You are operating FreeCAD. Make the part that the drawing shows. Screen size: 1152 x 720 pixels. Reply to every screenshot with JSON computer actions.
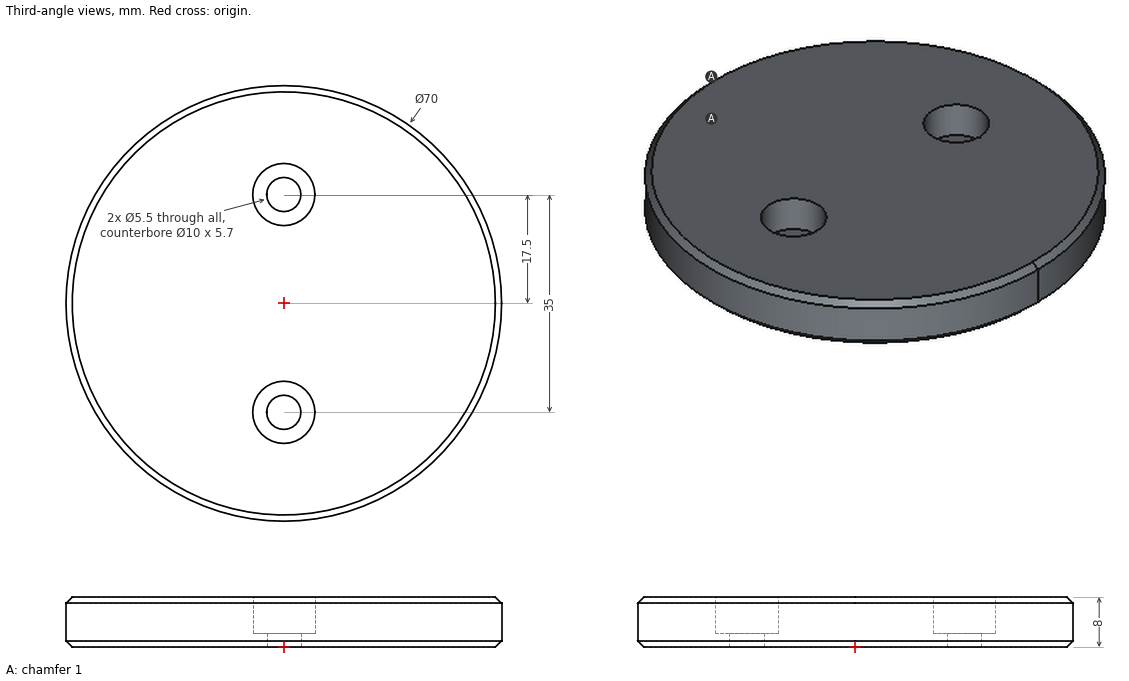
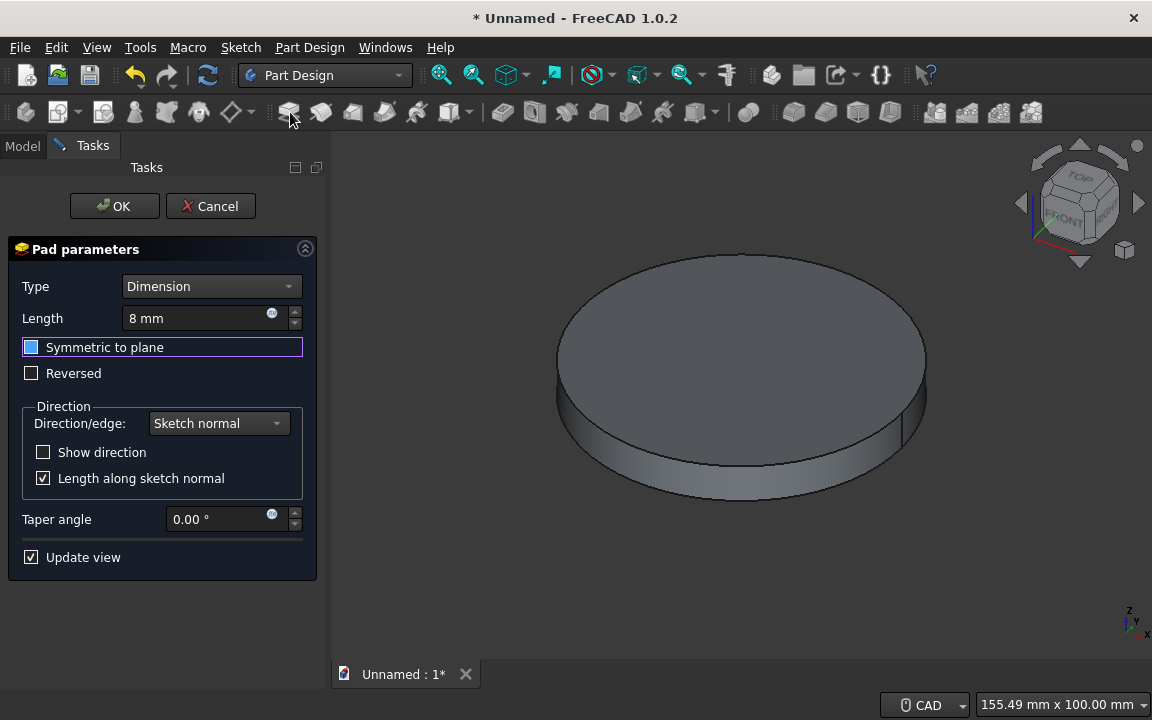
{"action": "left_click", "coordinate": [115, 206]}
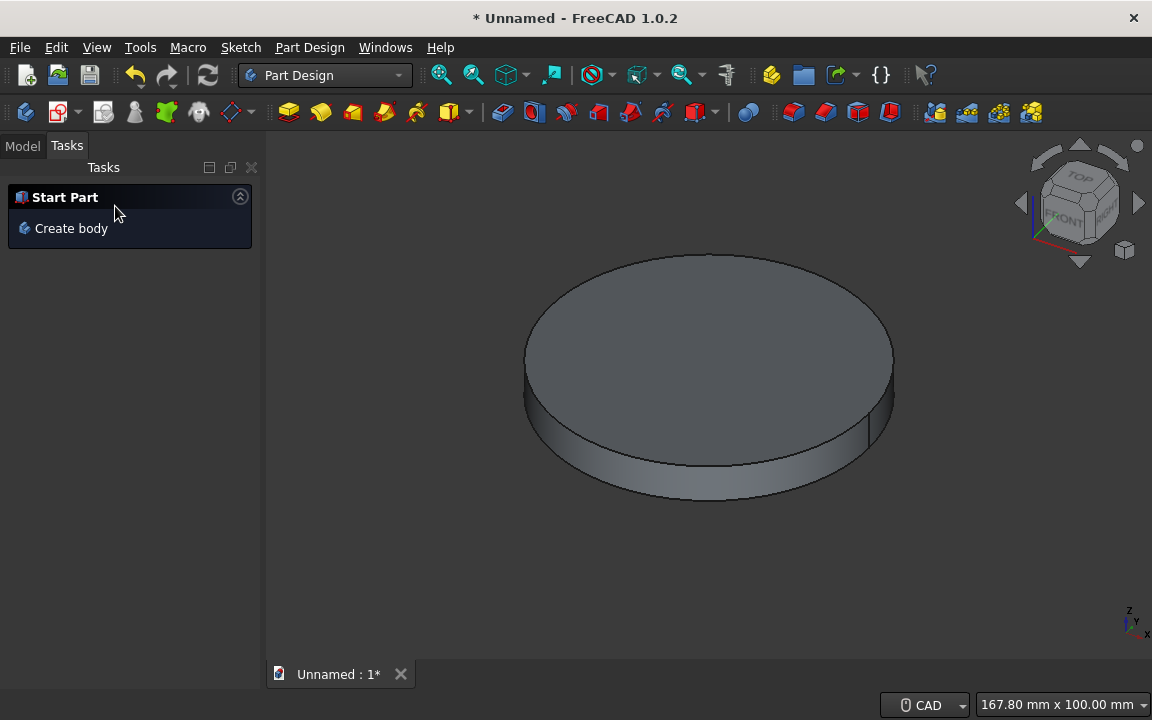
{"action": "left_click", "coordinate": [709, 359]}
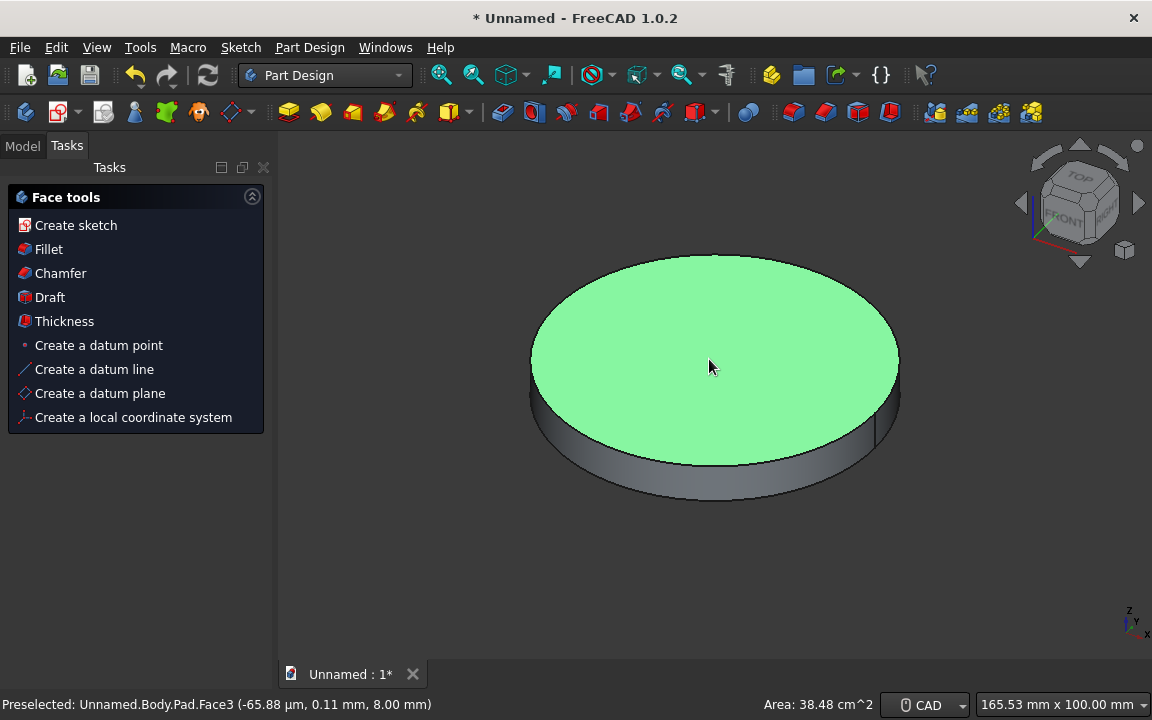
{"action": "left_click", "coordinate": [58, 112]}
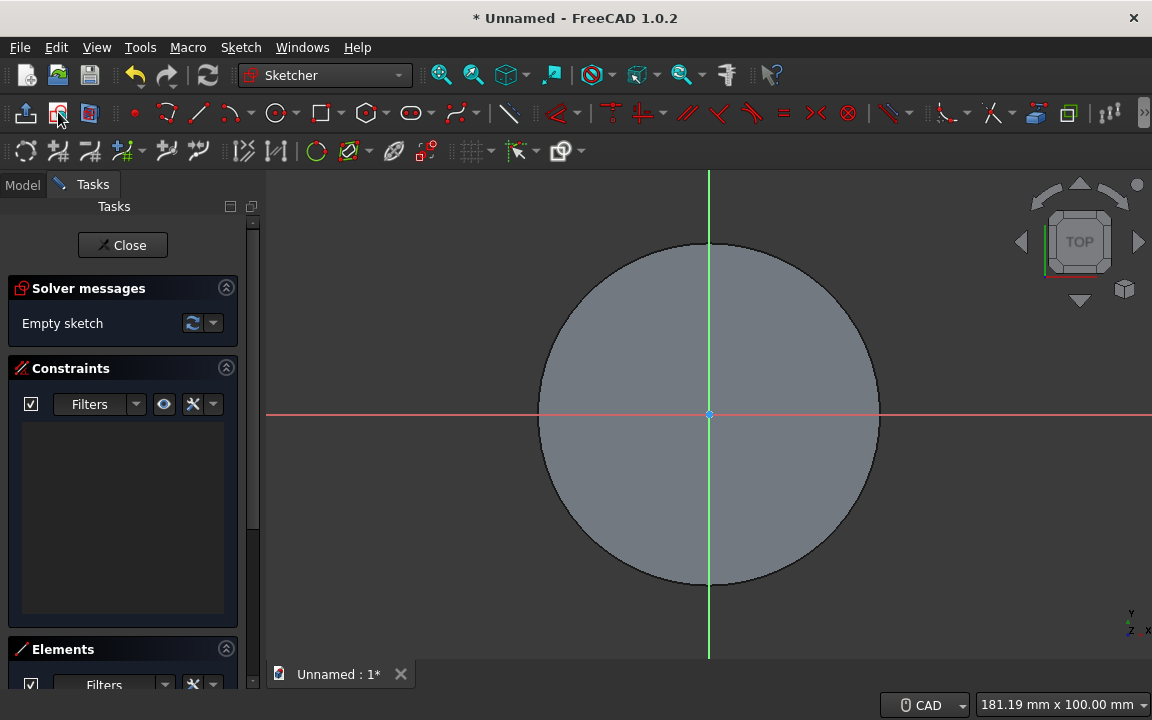
{"action": "scroll", "coordinate": [848, 414], "scroll_direction": "up", "scroll_amount": 2}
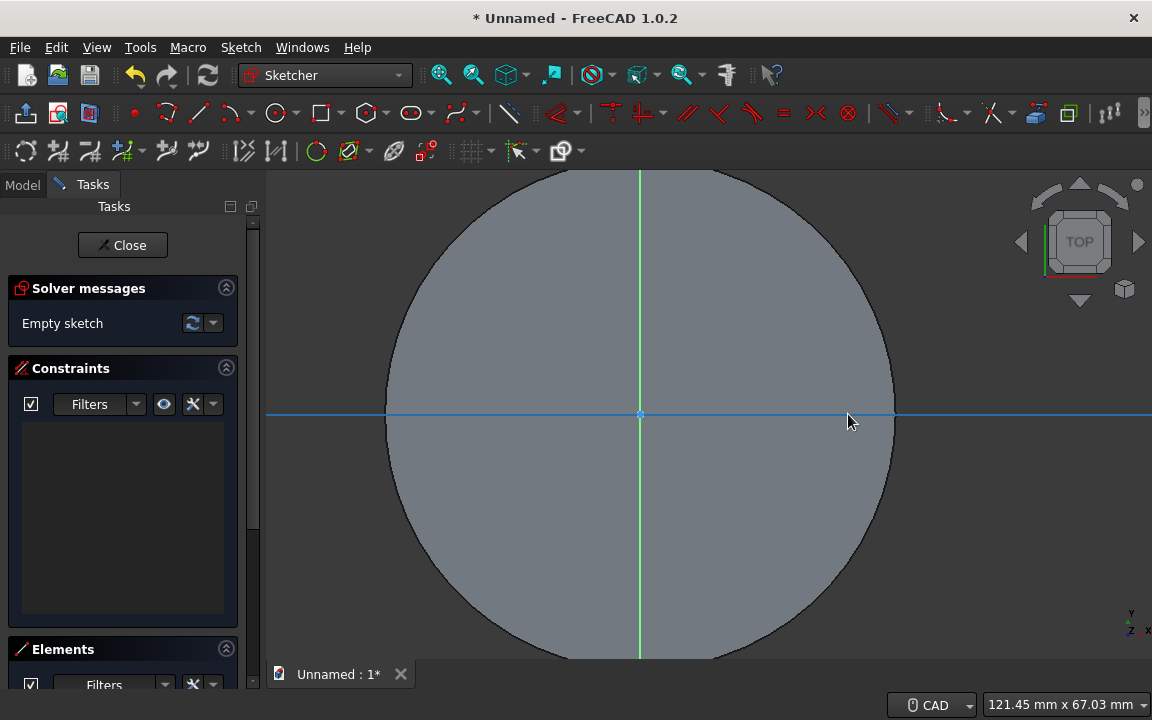
{"action": "left_click", "coordinate": [276, 114]}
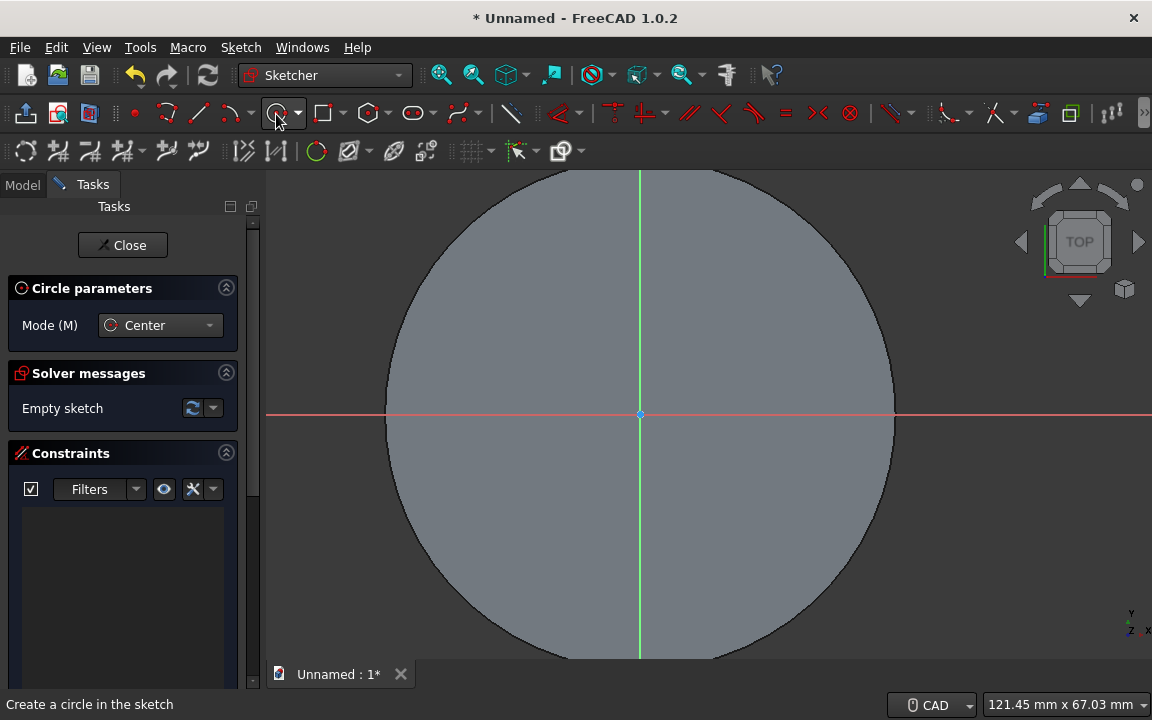
{"action": "left_click", "coordinate": [640, 287]}
{"action": "left_click", "coordinate": [654, 273]}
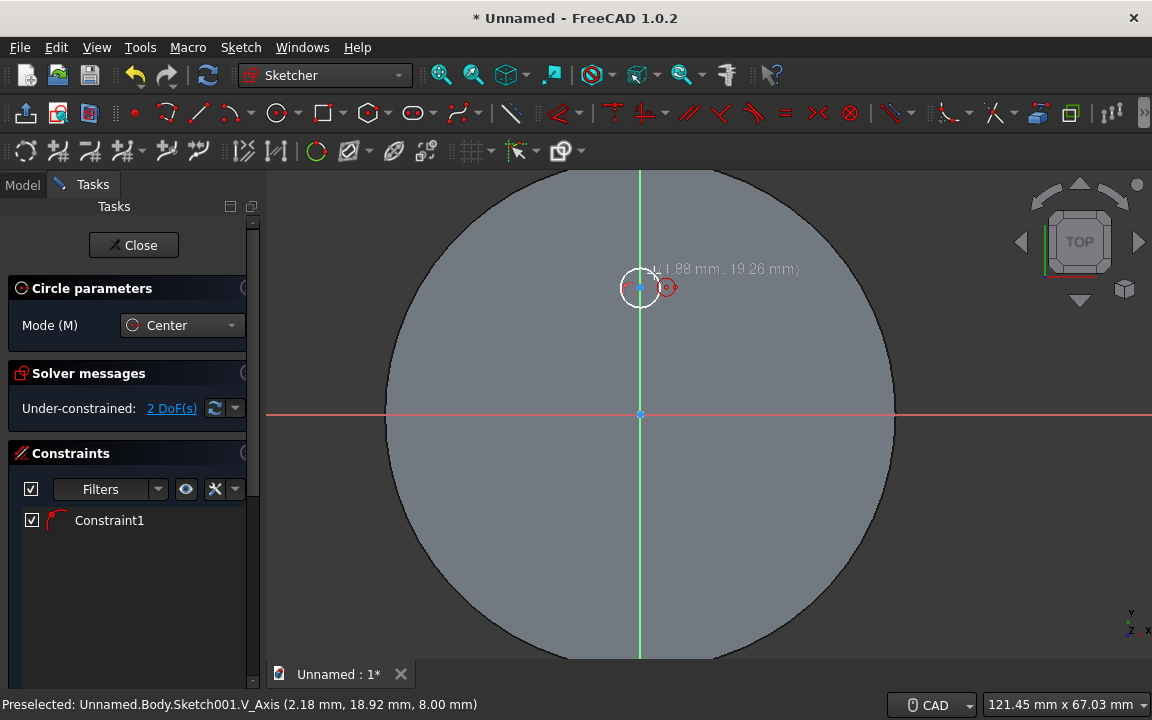
{"action": "left_click", "coordinate": [640, 542]}
{"action": "left_click", "coordinate": [654, 528]}
{"action": "key", "text": "Escape"}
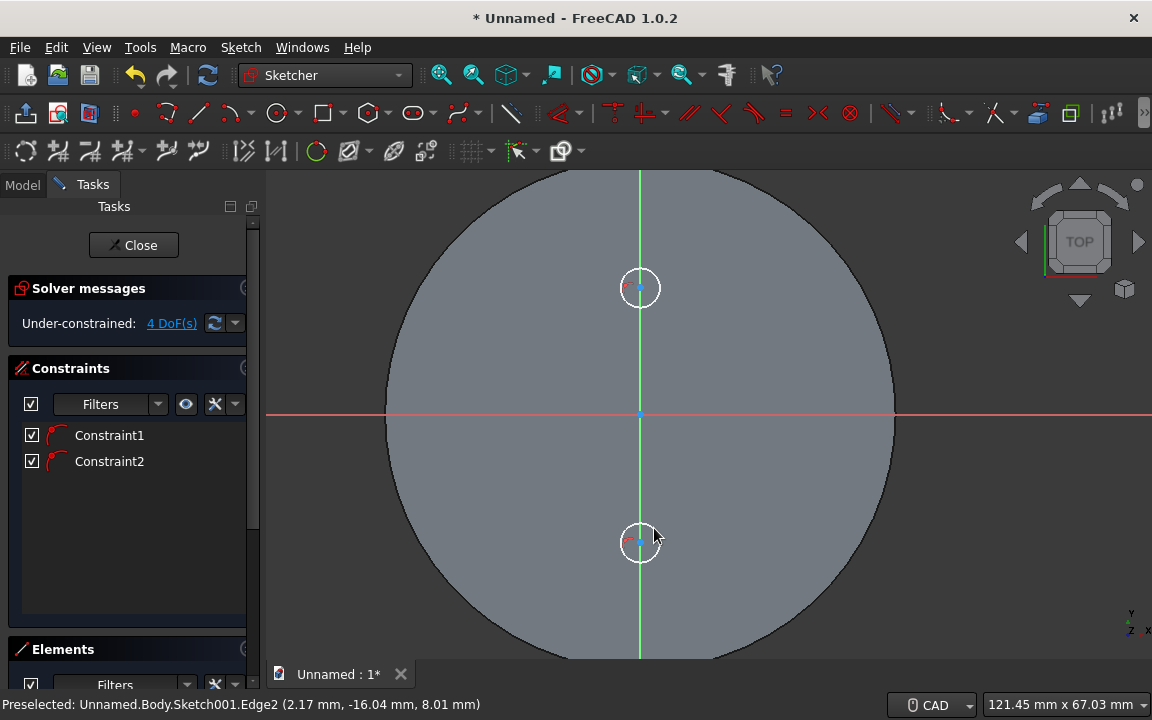
{"action": "left_click", "coordinate": [654, 274]}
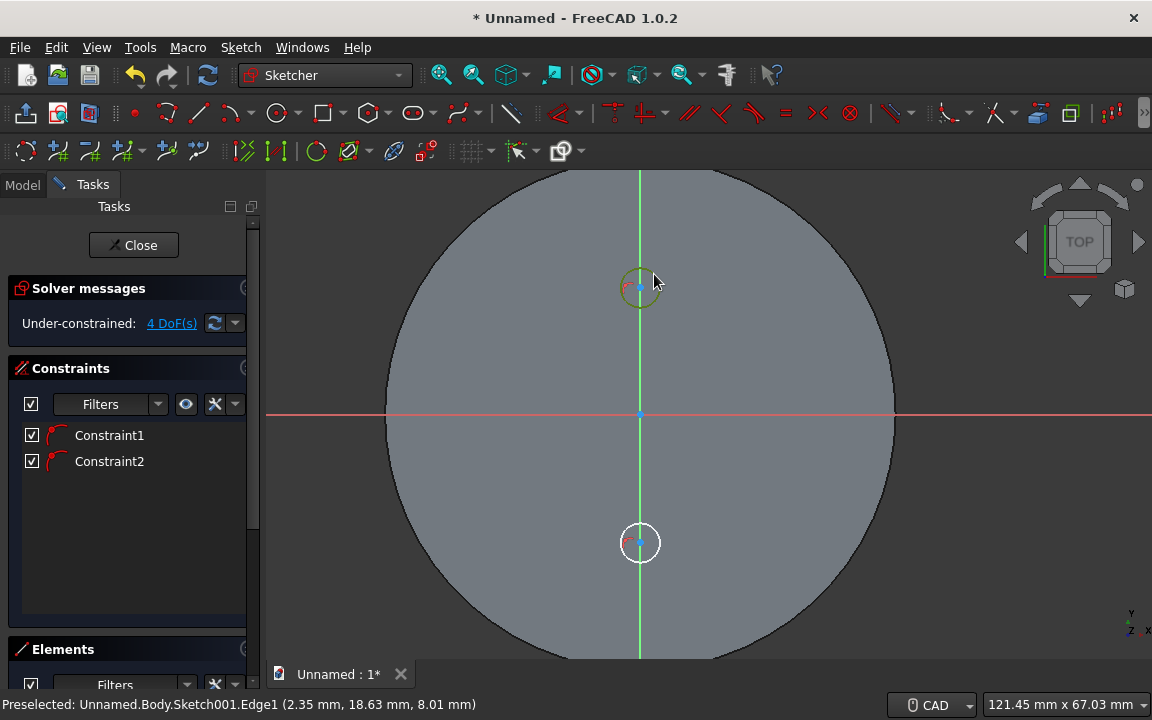
{"action": "left_click", "coordinate": [654, 529]}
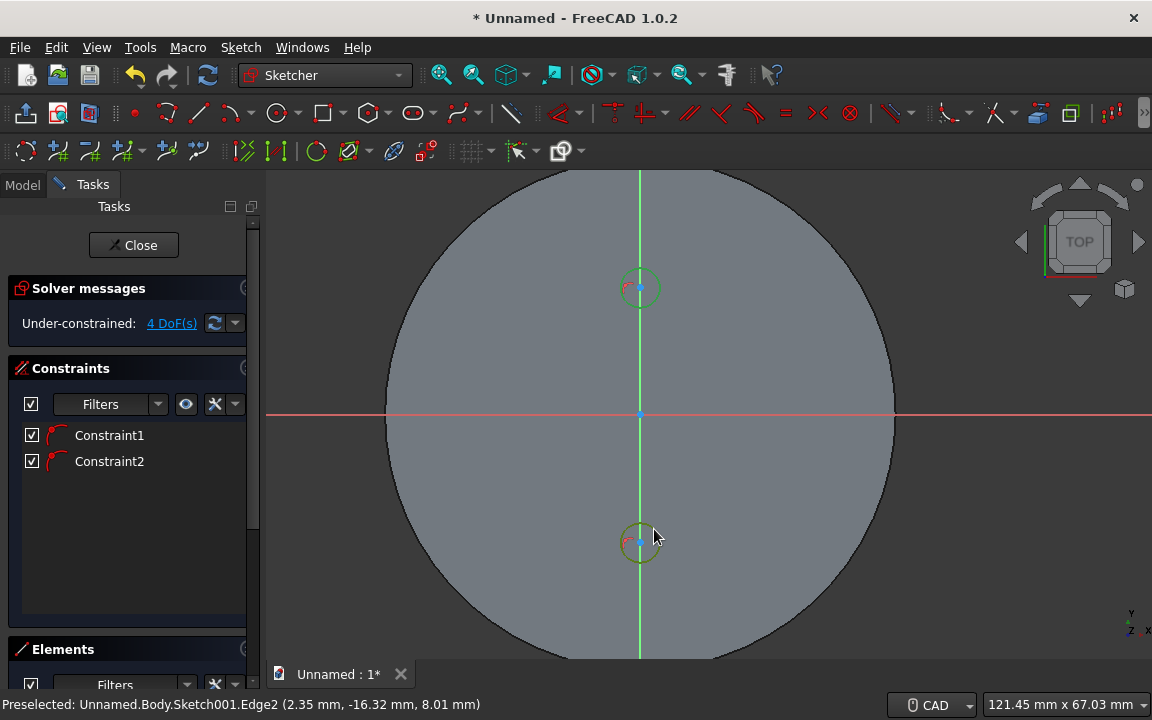
{"action": "key", "text": "e"}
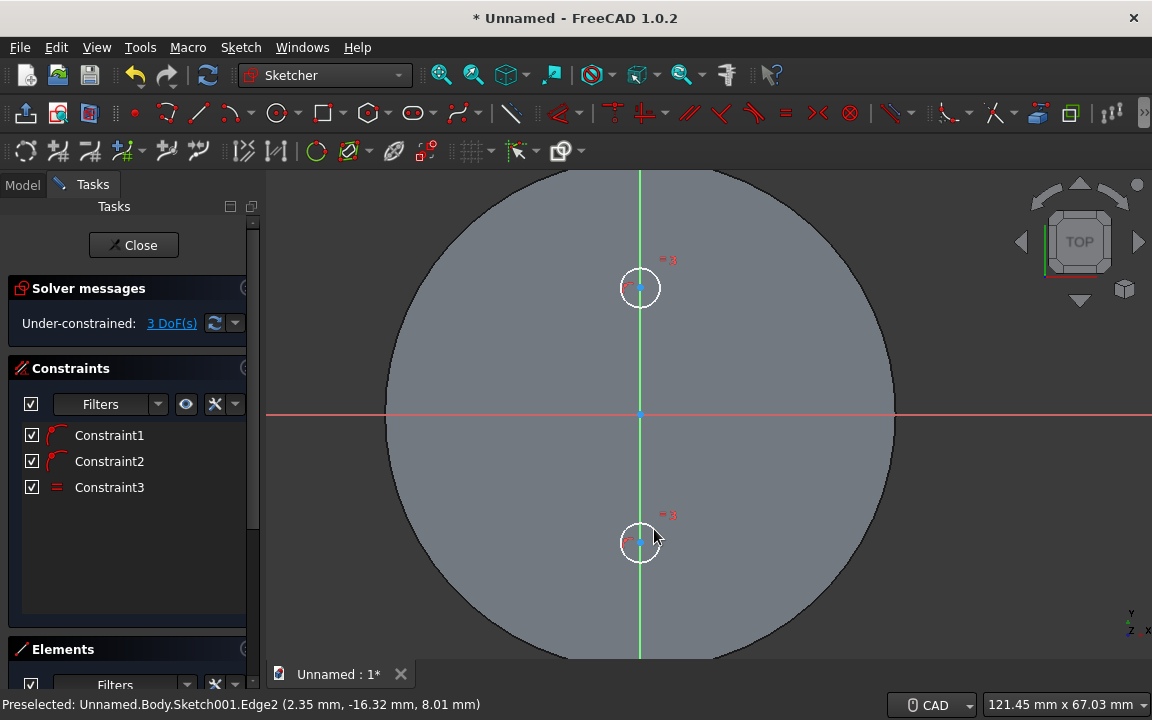
{"action": "left_click", "coordinate": [558, 114]}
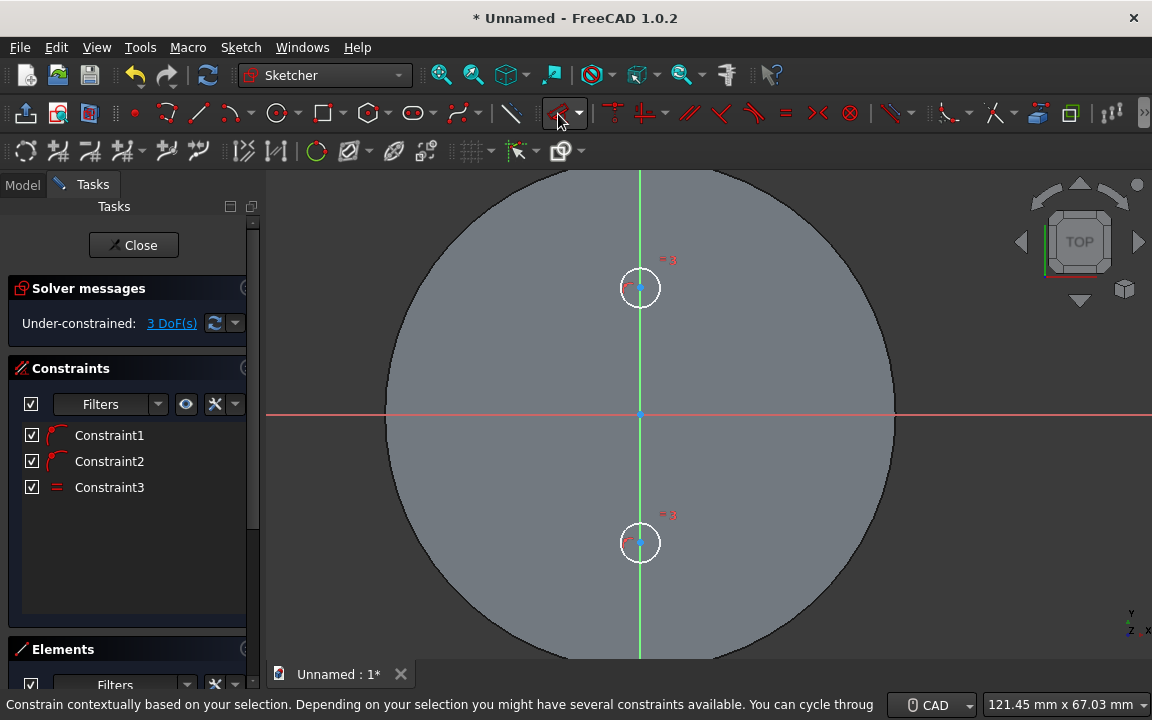
{"action": "left_click", "coordinate": [654, 274]}
{"action": "left_click", "coordinate": [676, 251]}